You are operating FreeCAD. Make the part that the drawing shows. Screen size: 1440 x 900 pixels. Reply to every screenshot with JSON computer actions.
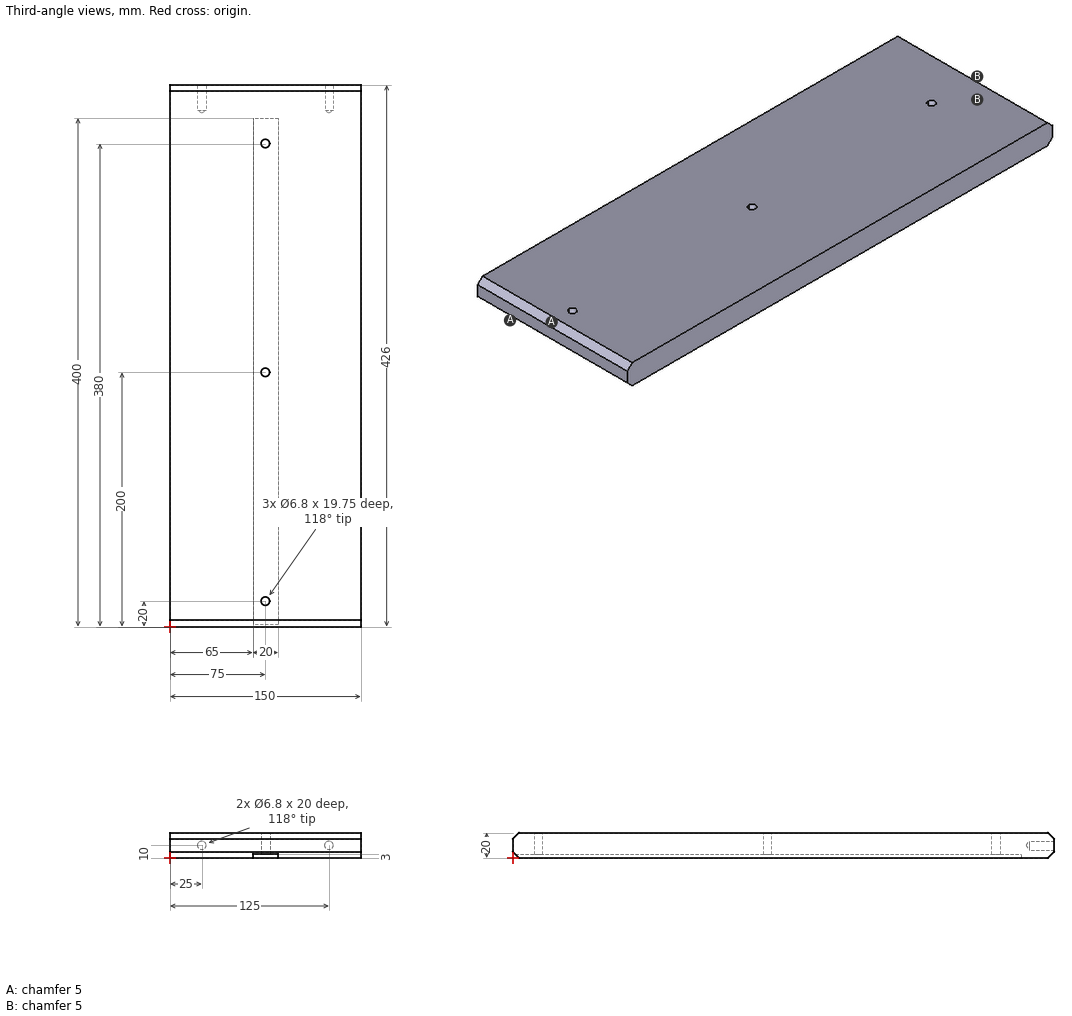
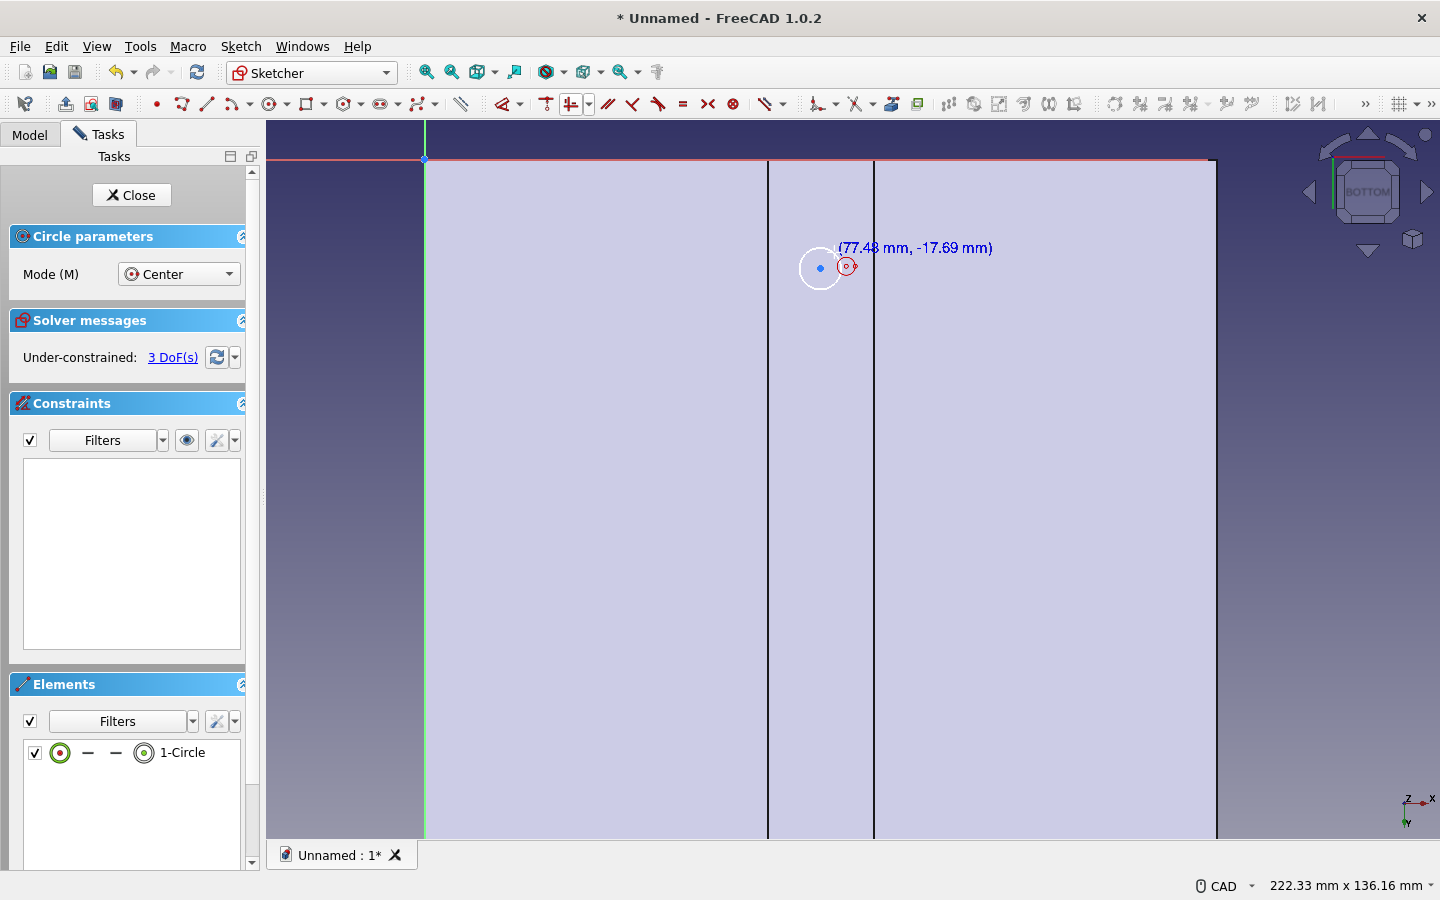
{"action": "scroll", "coordinate": [834, 253], "scroll_direction": "down", "scroll_amount": 7}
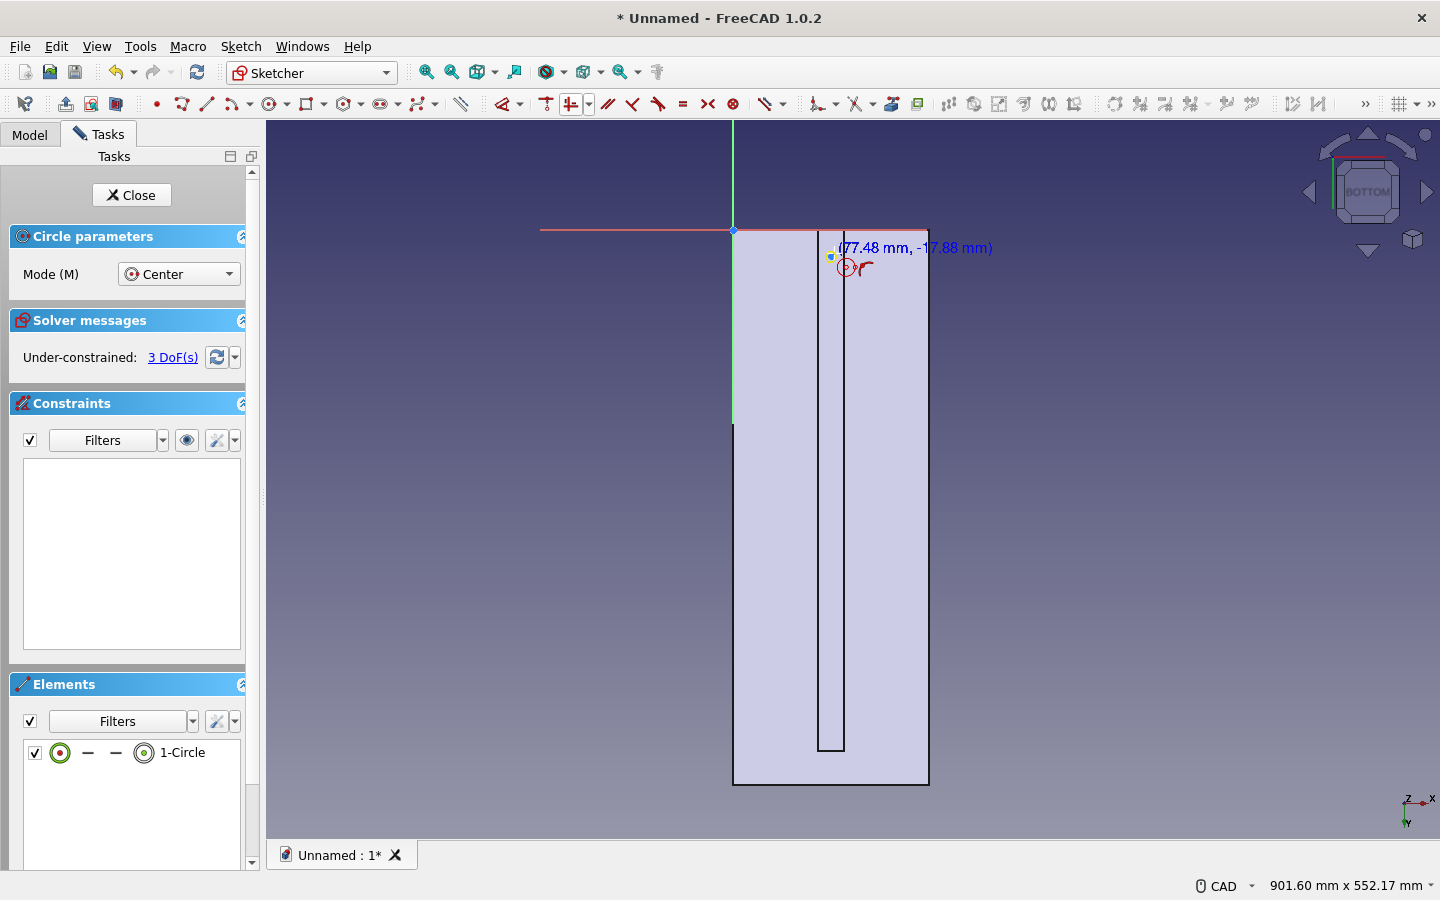
{"action": "scroll", "coordinate": [831, 491], "scroll_direction": "up", "scroll_amount": 9}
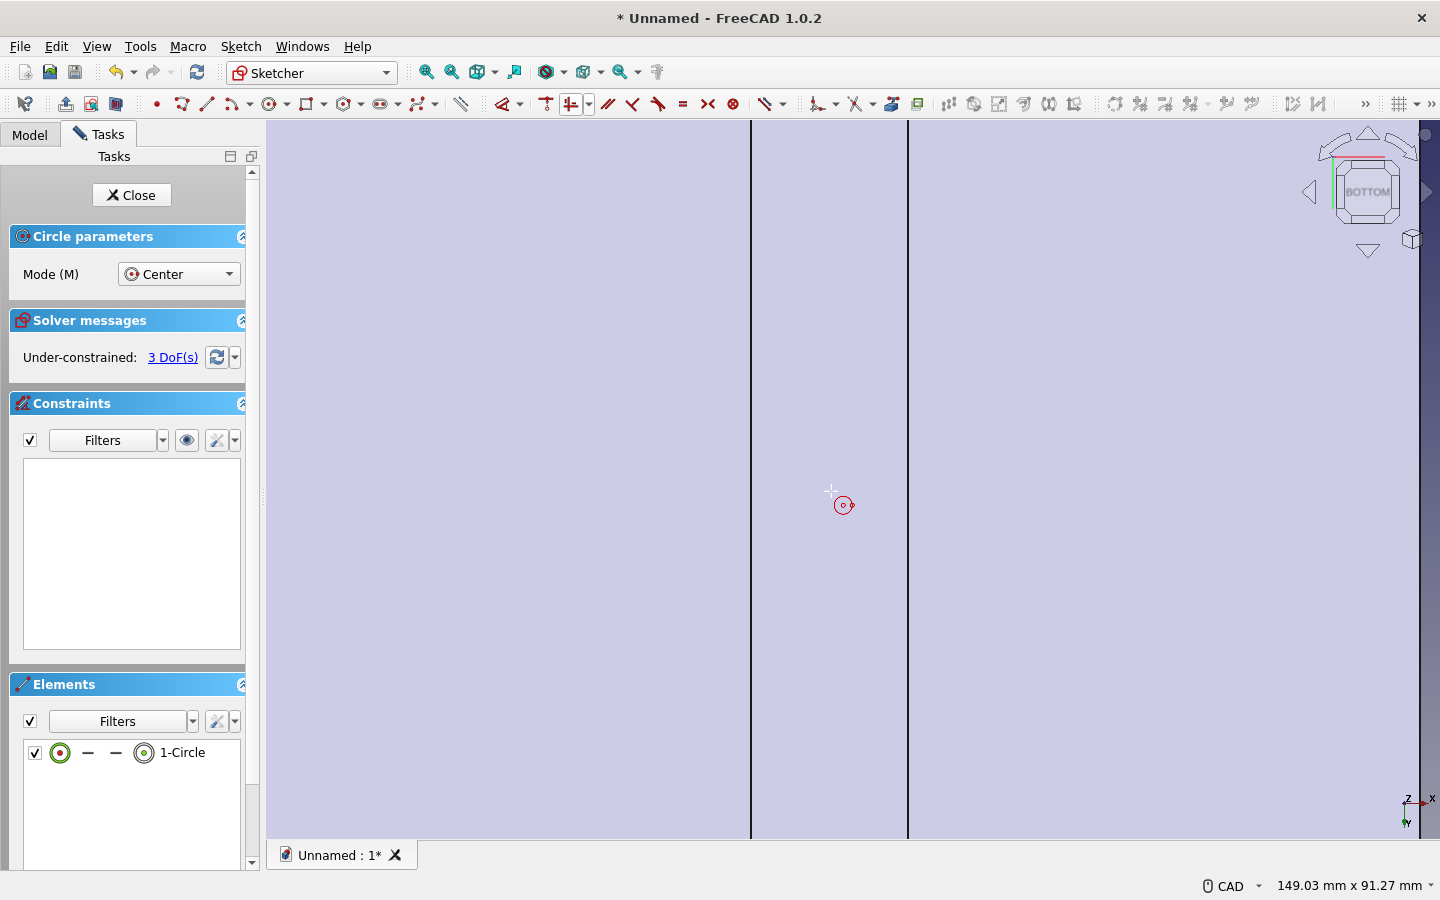
{"action": "scroll", "coordinate": [831, 491], "scroll_direction": "down", "scroll_amount": 9}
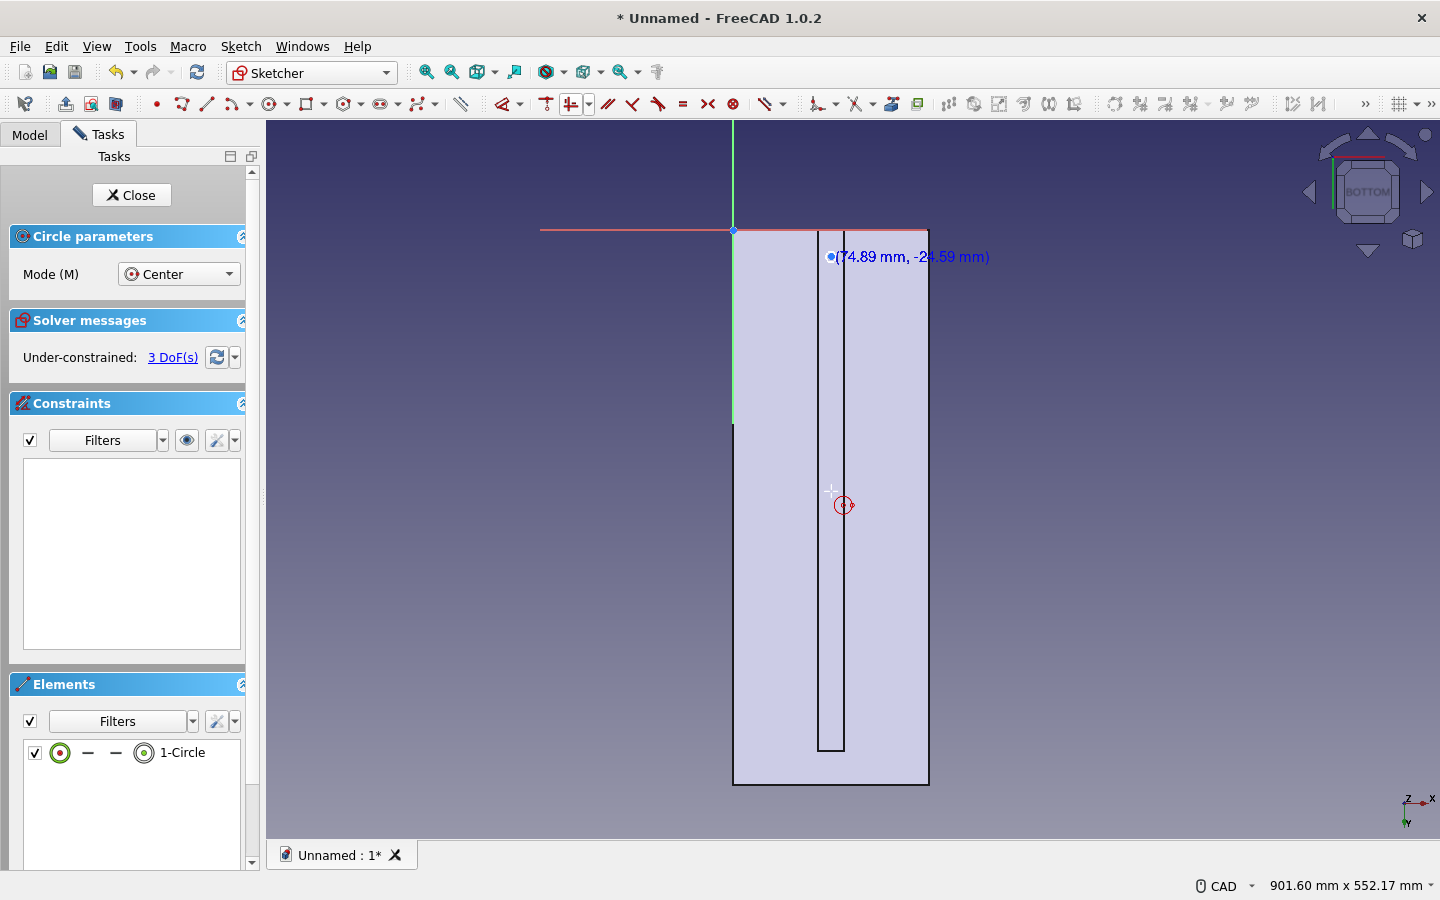
{"action": "left_click", "coordinate": [831, 491]}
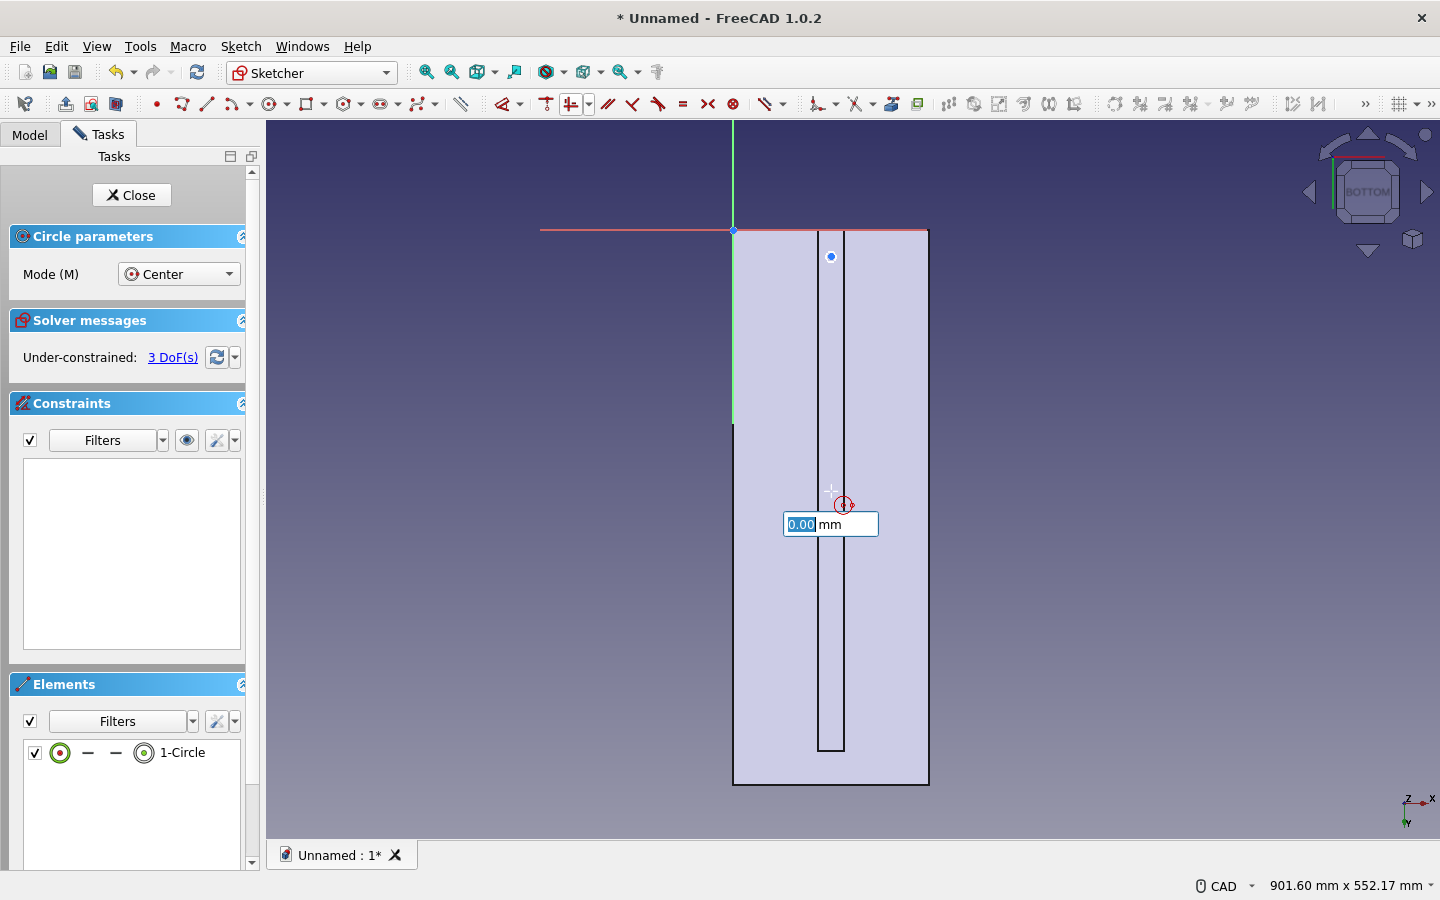
{"action": "scroll", "coordinate": [834, 487], "scroll_direction": "up", "scroll_amount": 7}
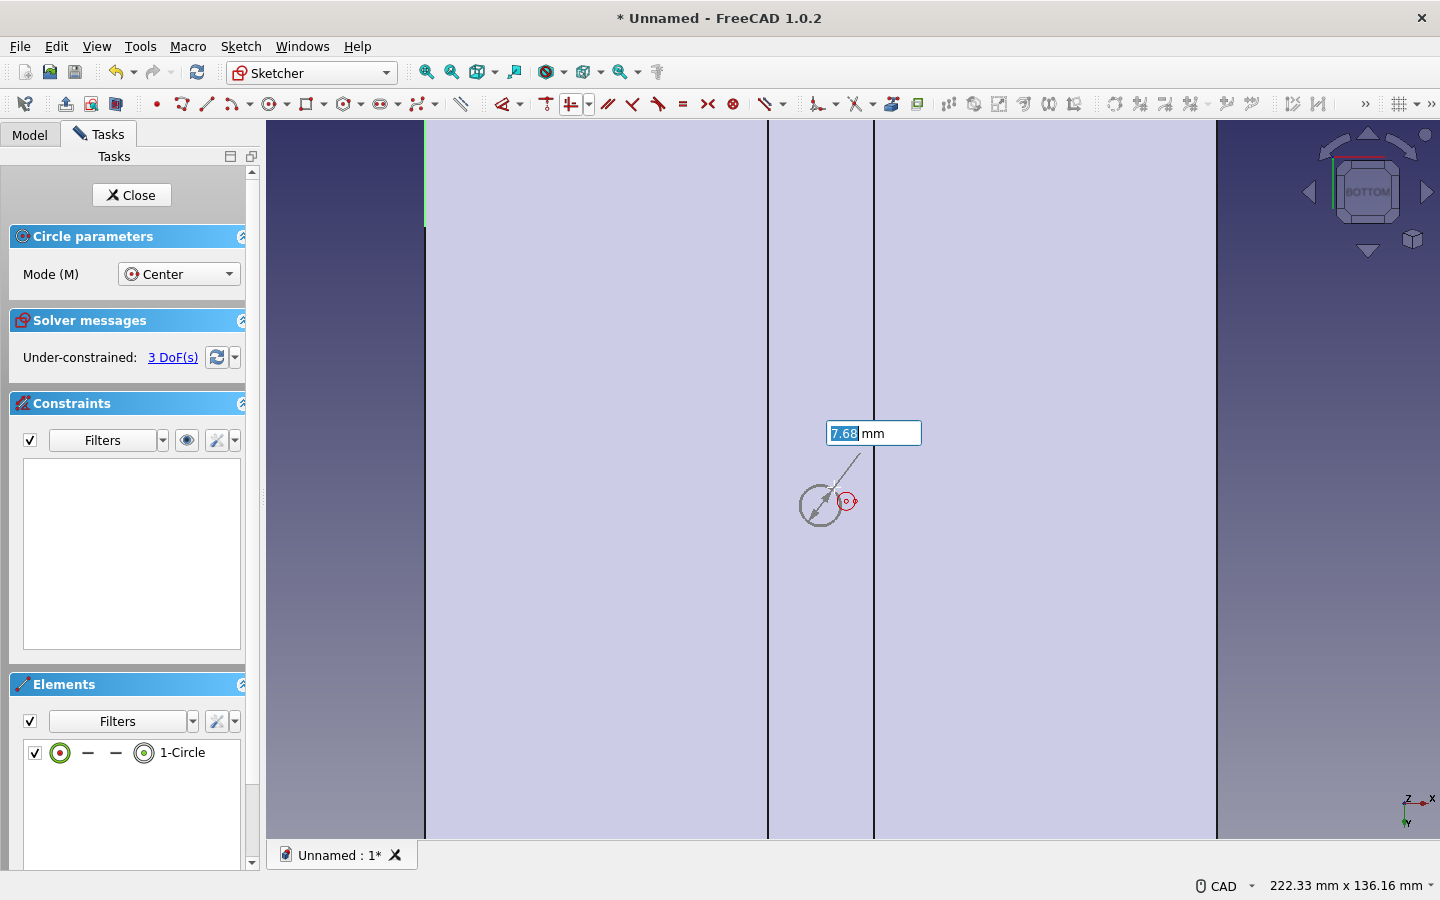
{"action": "left_click", "coordinate": [834, 487]}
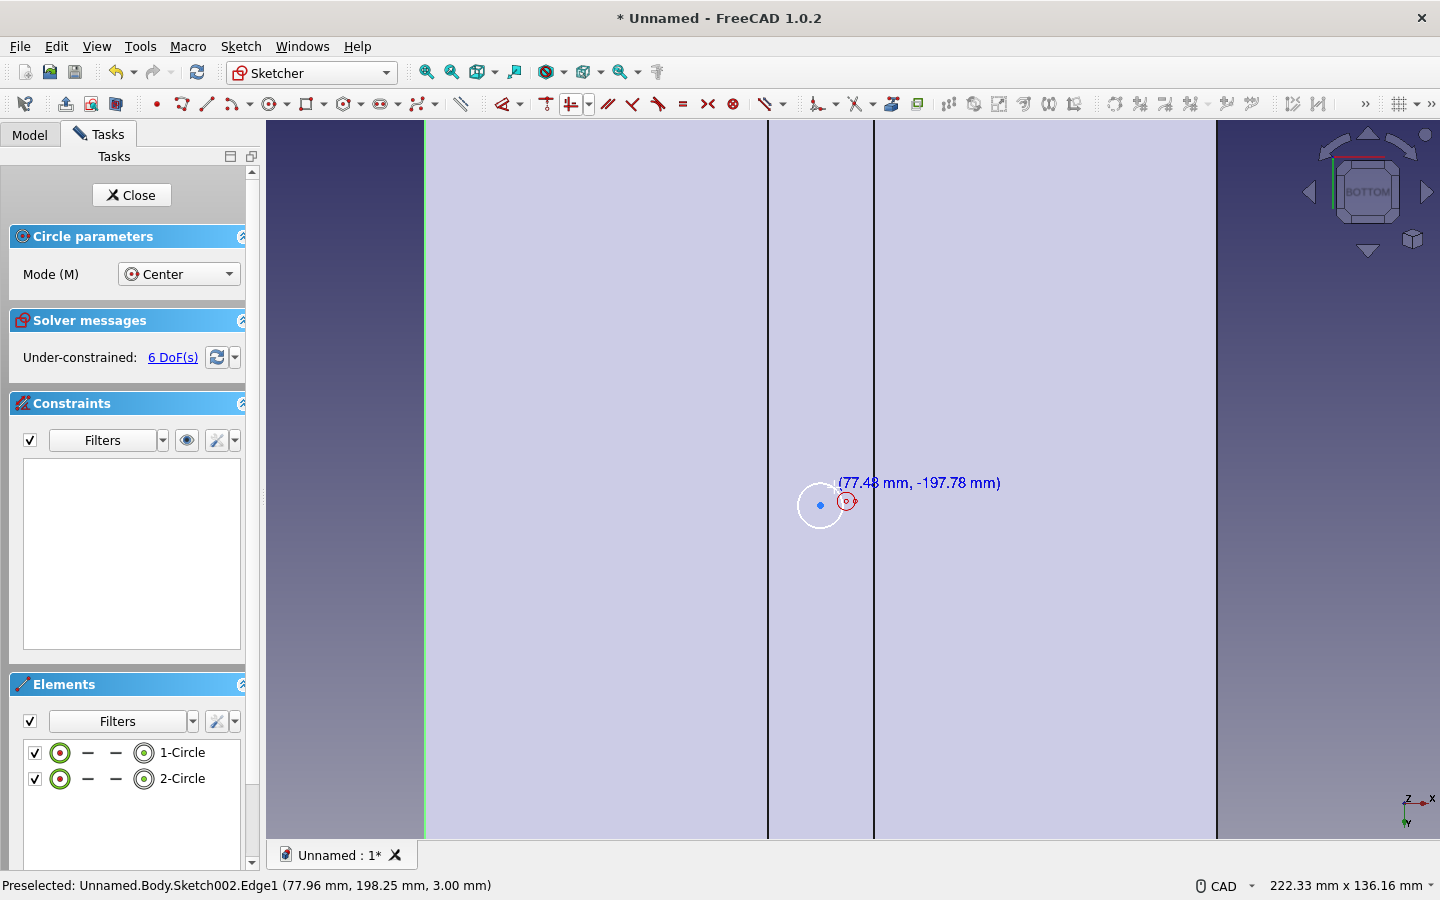
{"action": "scroll", "coordinate": [834, 487], "scroll_direction": "down", "scroll_amount": 7}